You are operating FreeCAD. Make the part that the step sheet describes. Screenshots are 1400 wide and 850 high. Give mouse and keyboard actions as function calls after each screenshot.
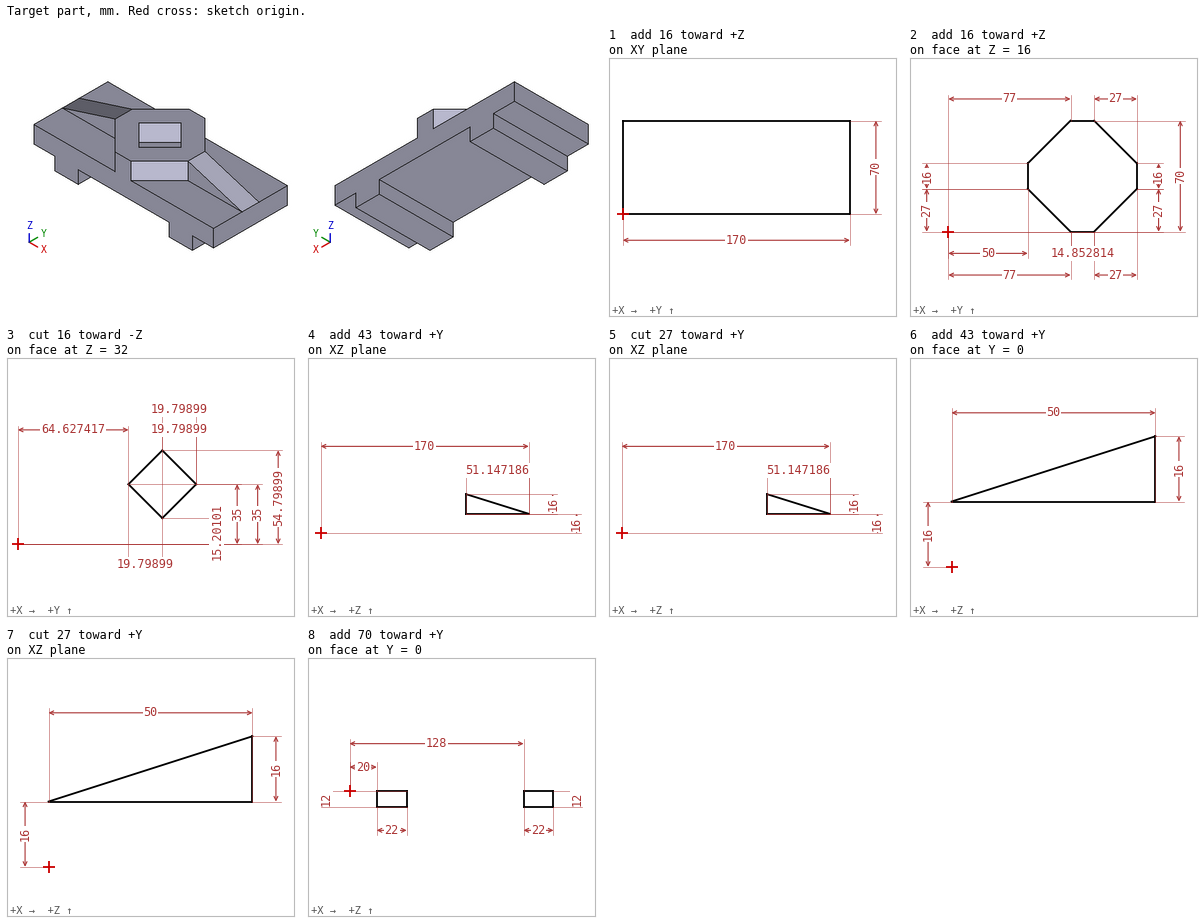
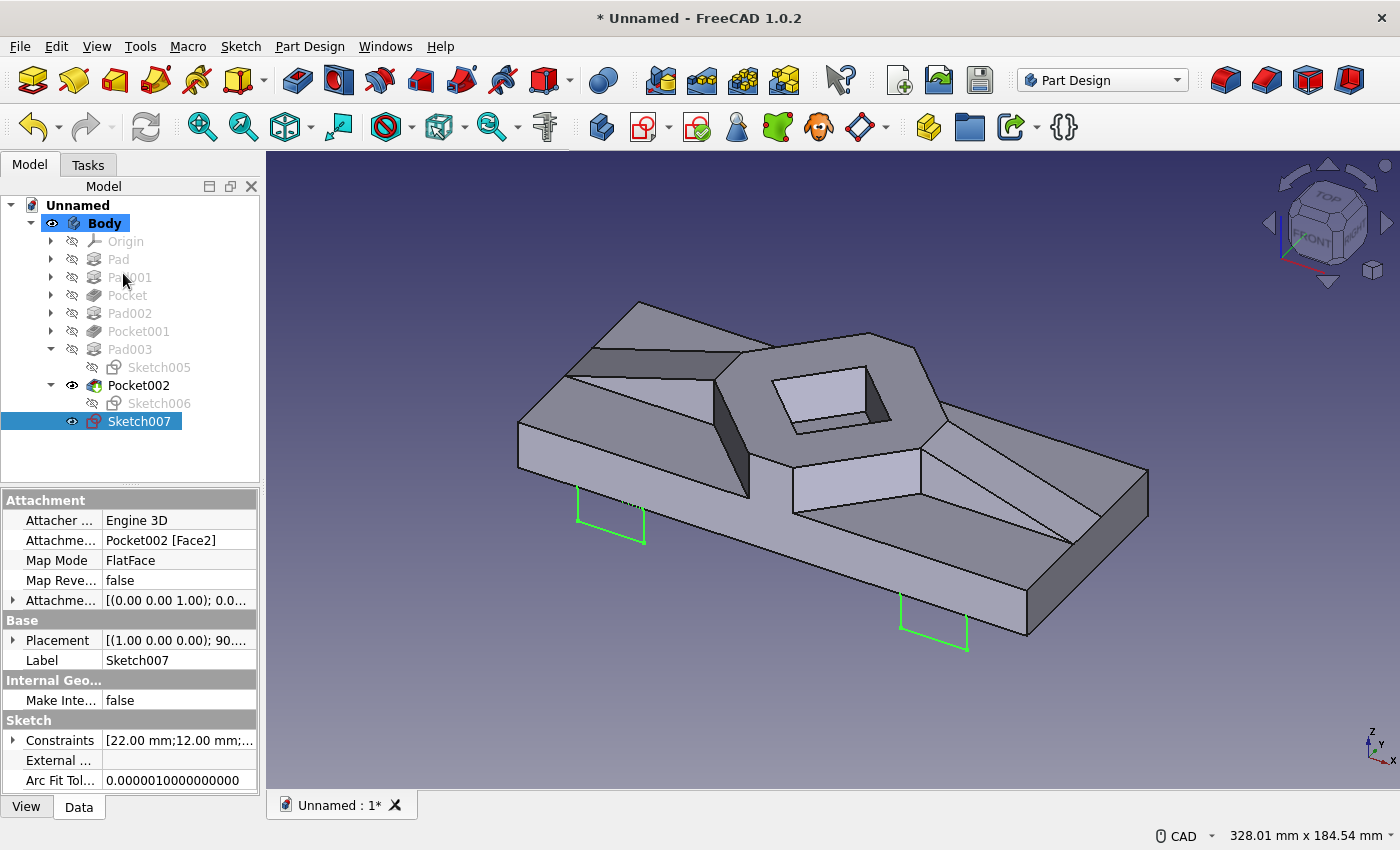
click(33, 80)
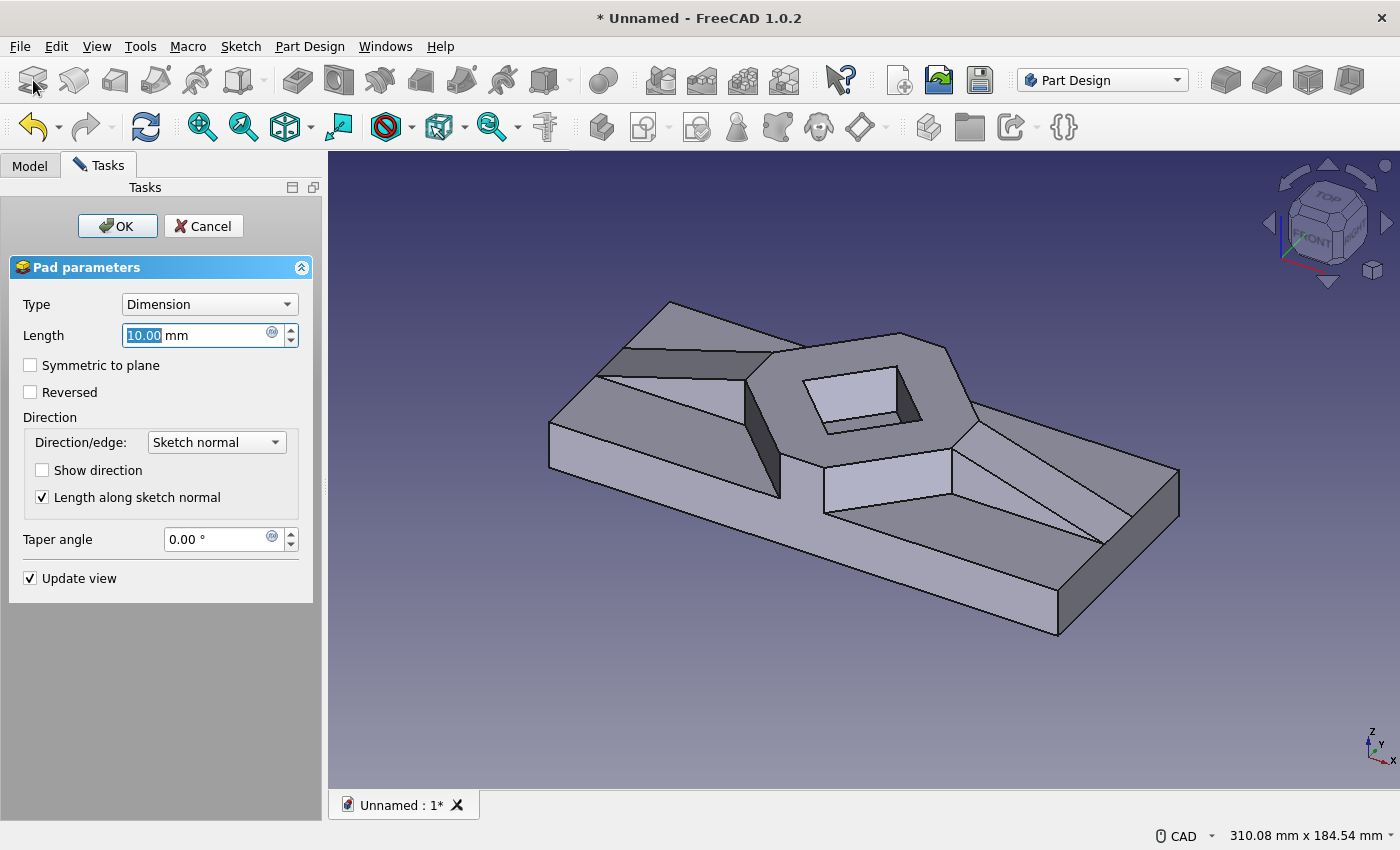
text(70)
key(Tab)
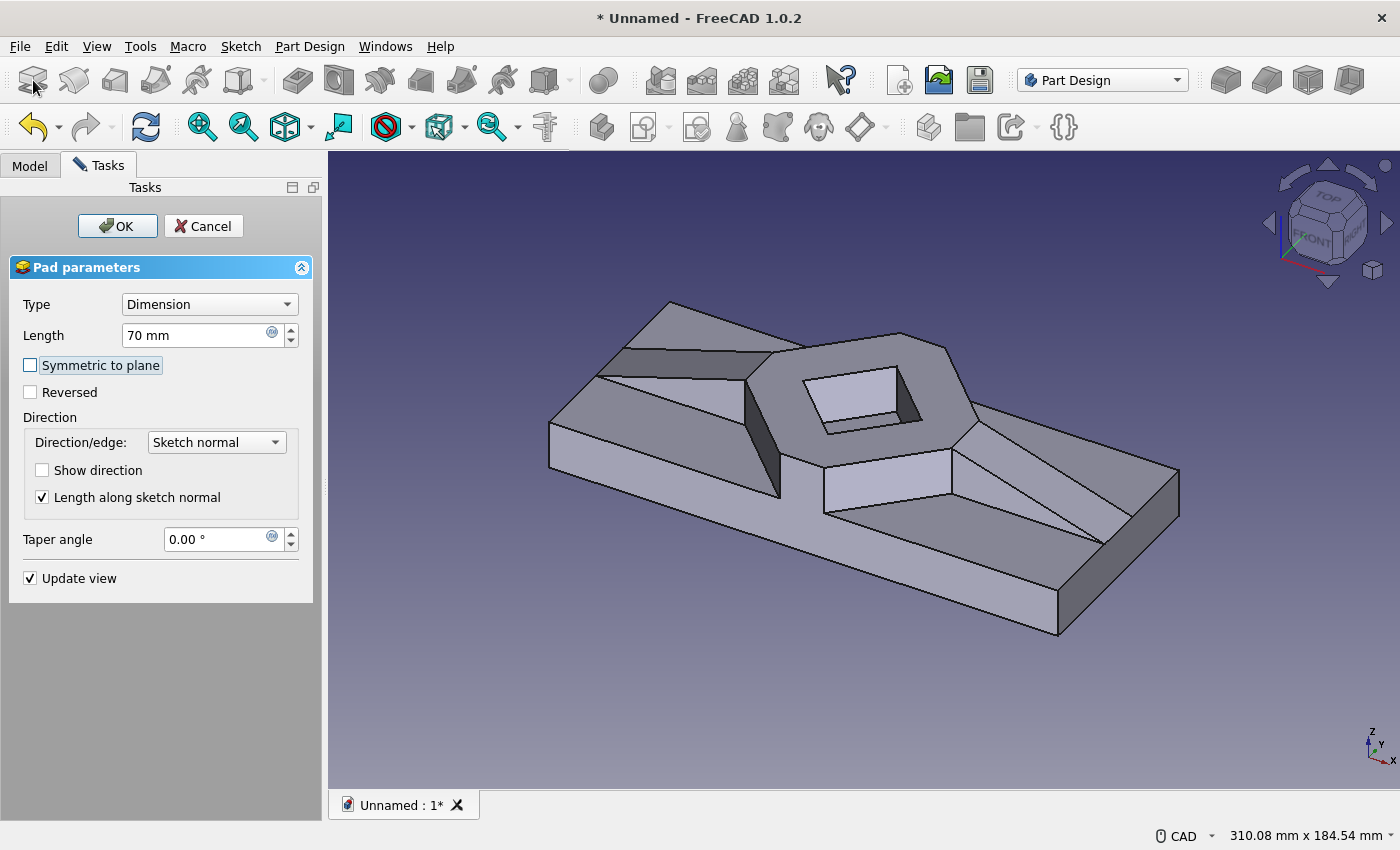
click(31, 392)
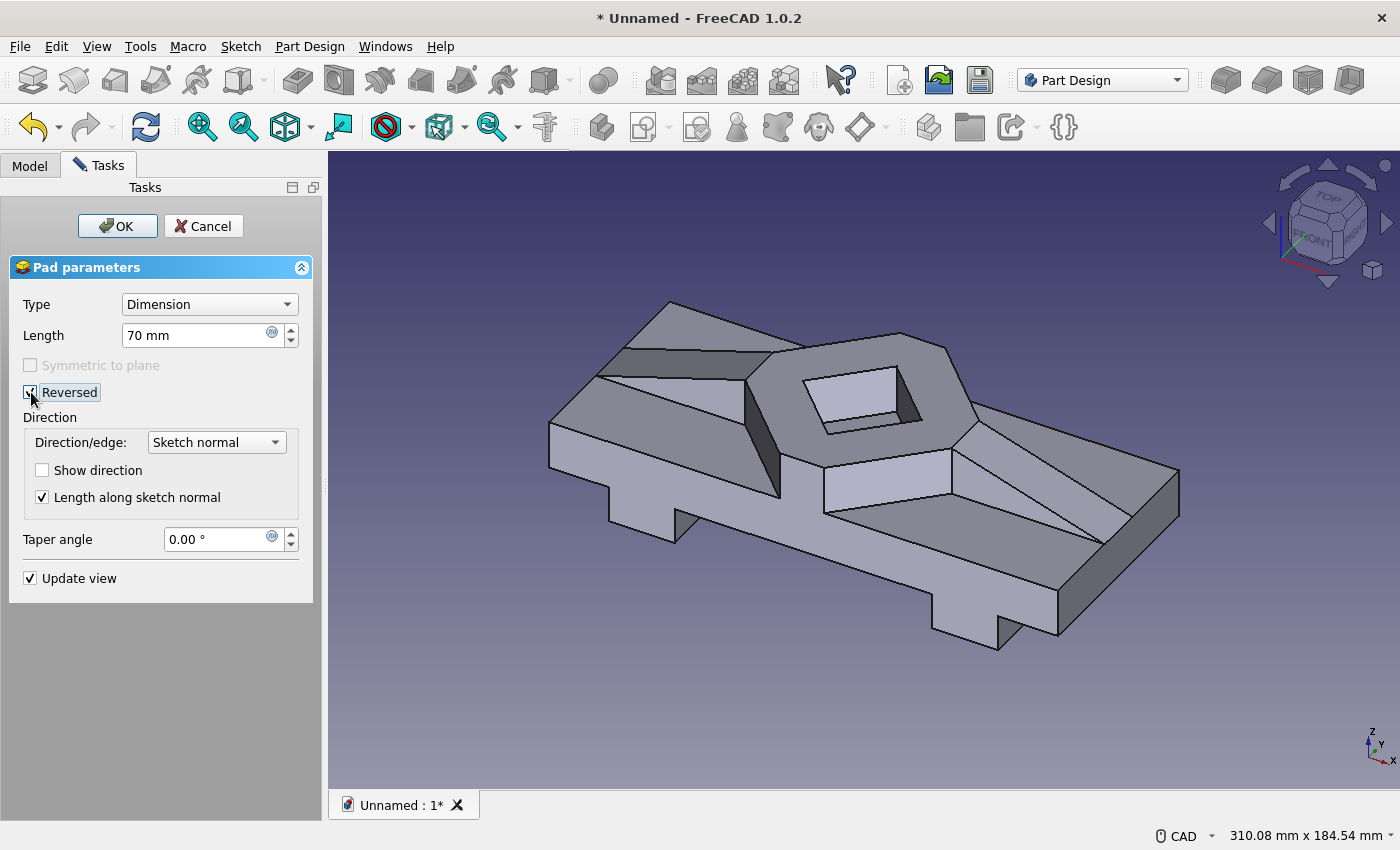
click(118, 226)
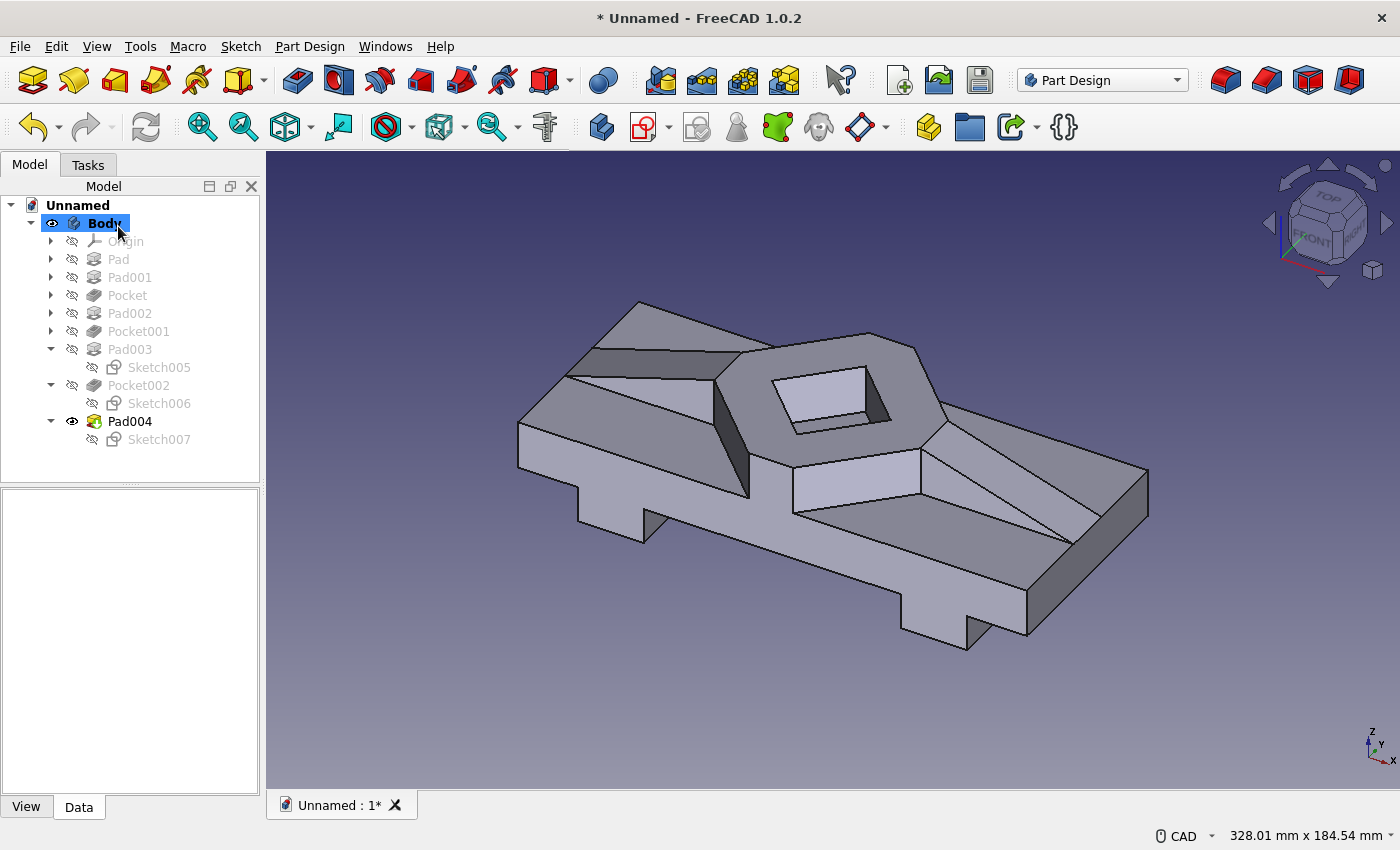
key(0)